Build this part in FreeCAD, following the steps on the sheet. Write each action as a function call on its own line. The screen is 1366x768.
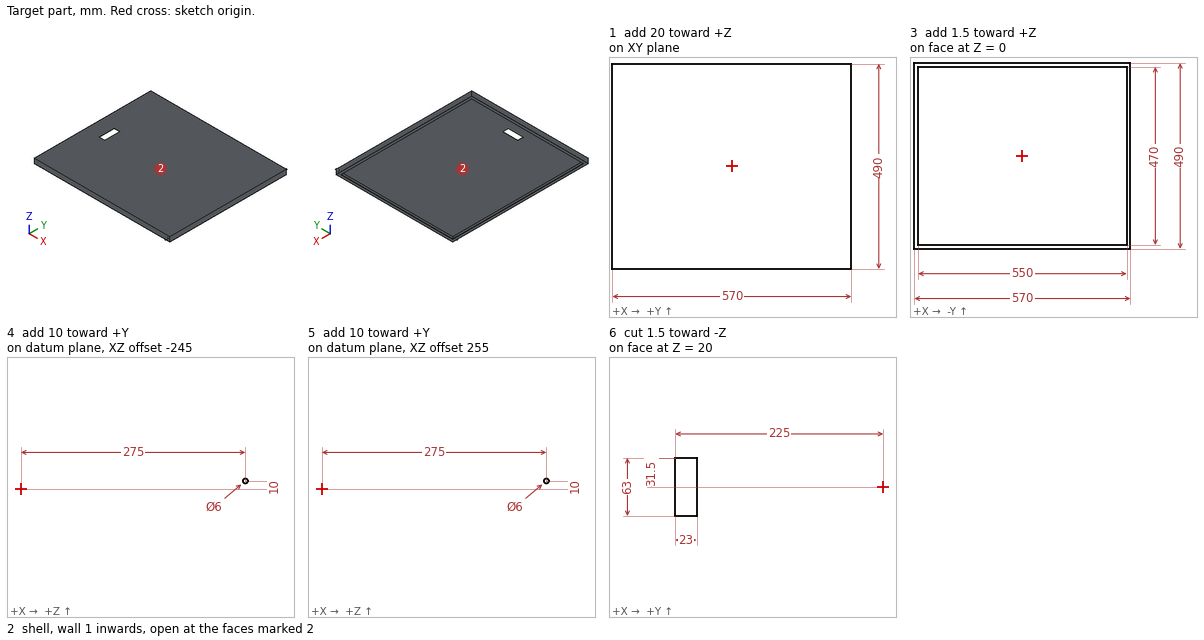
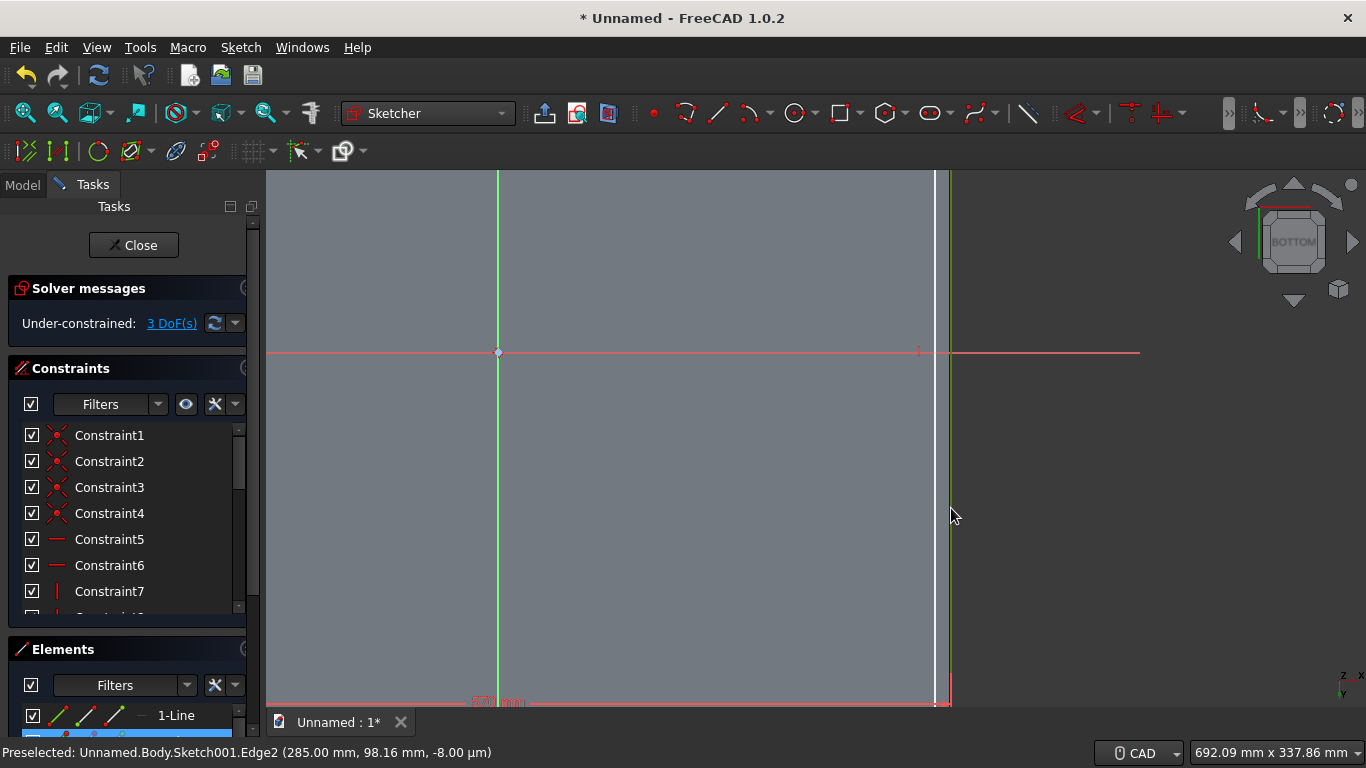
key(i)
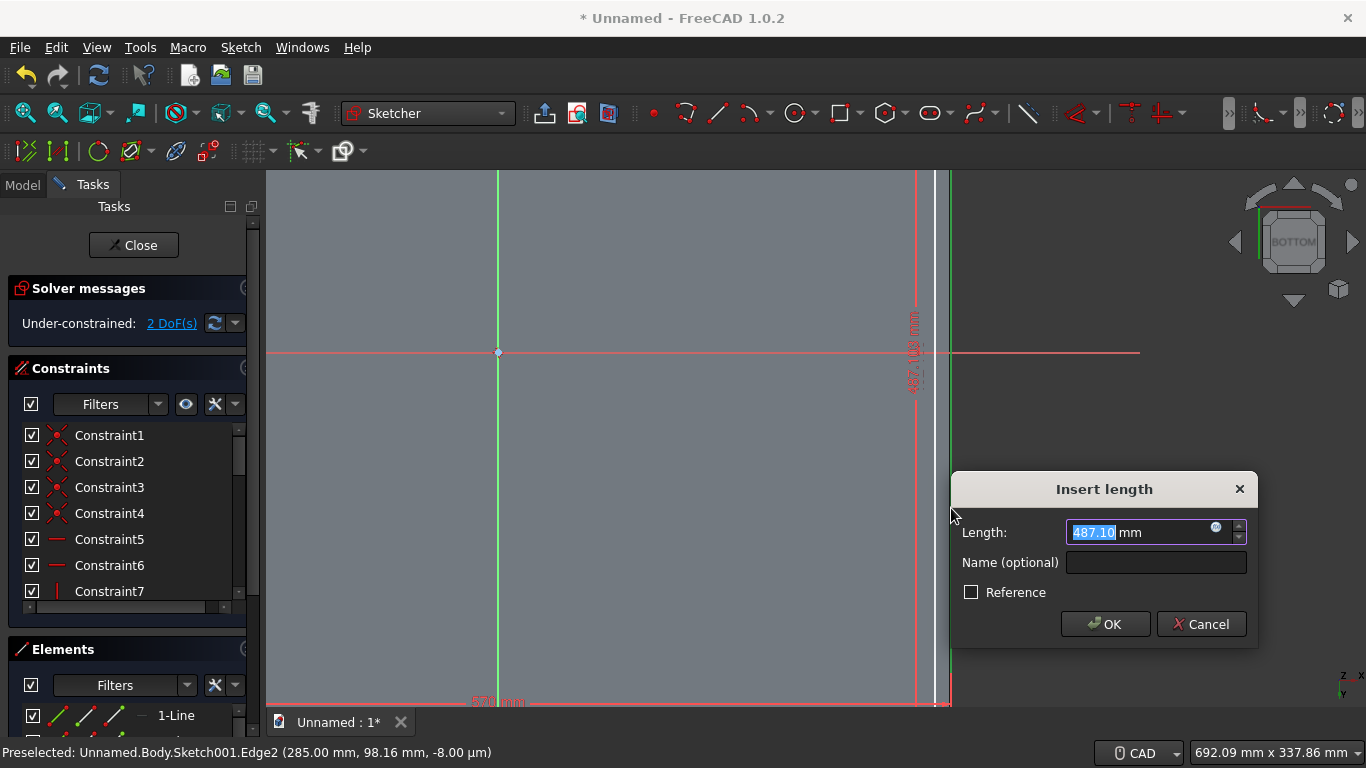
text(490)
key(Return)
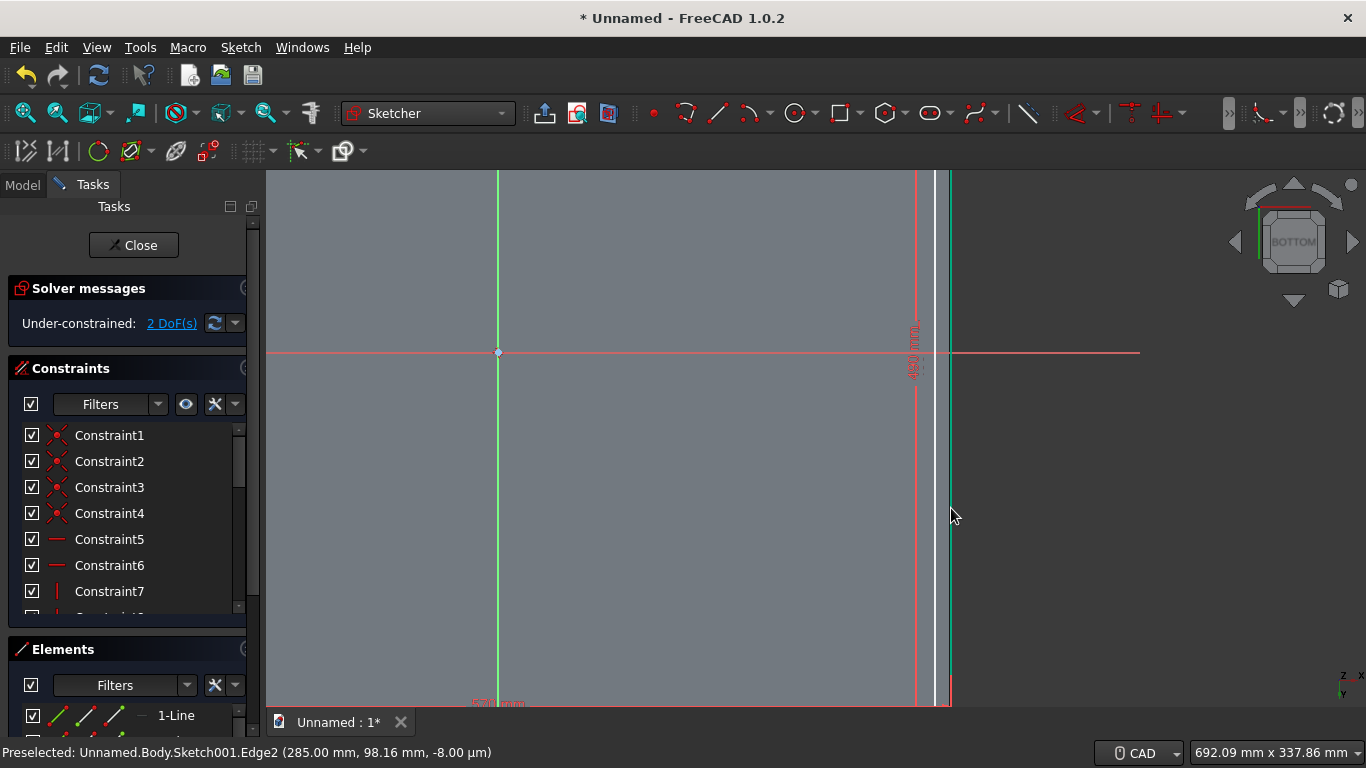
scroll(951, 508, down, 4)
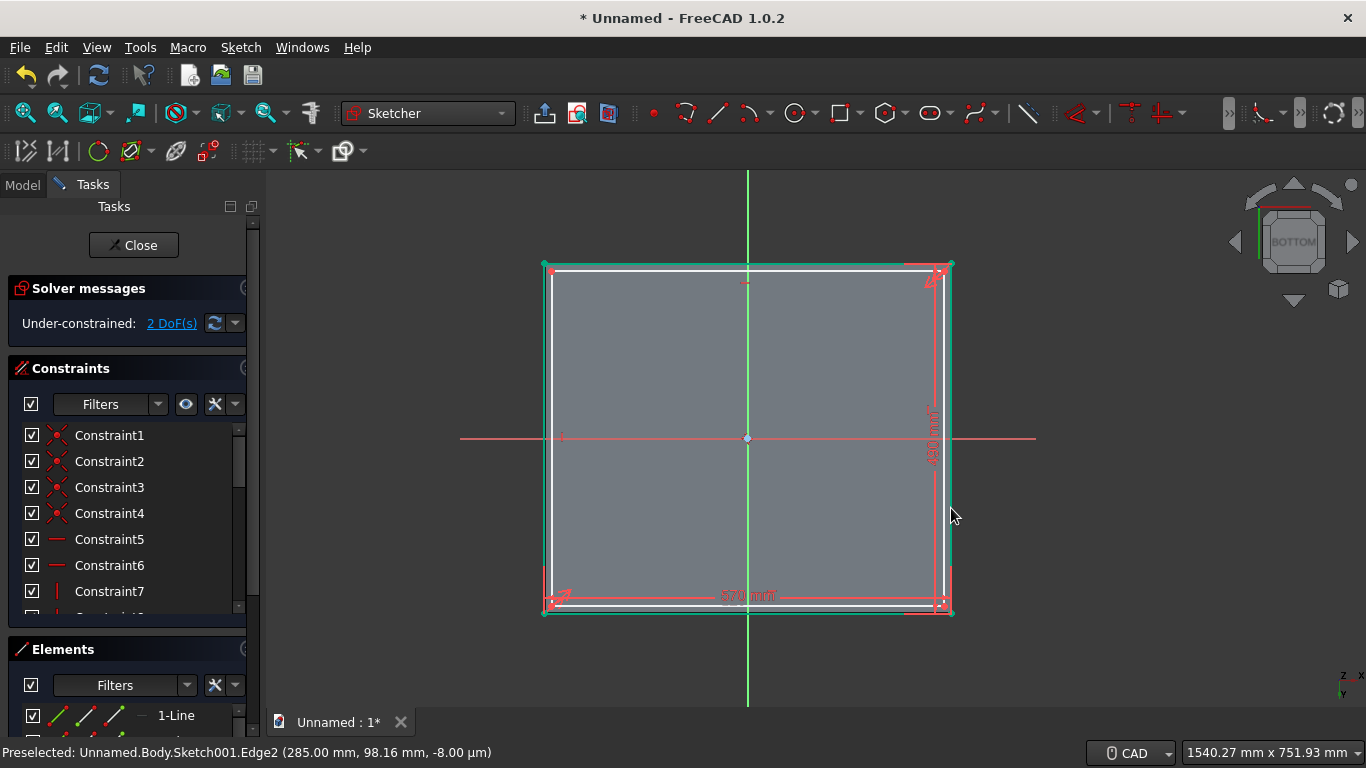
scroll(669, 606, up, 4)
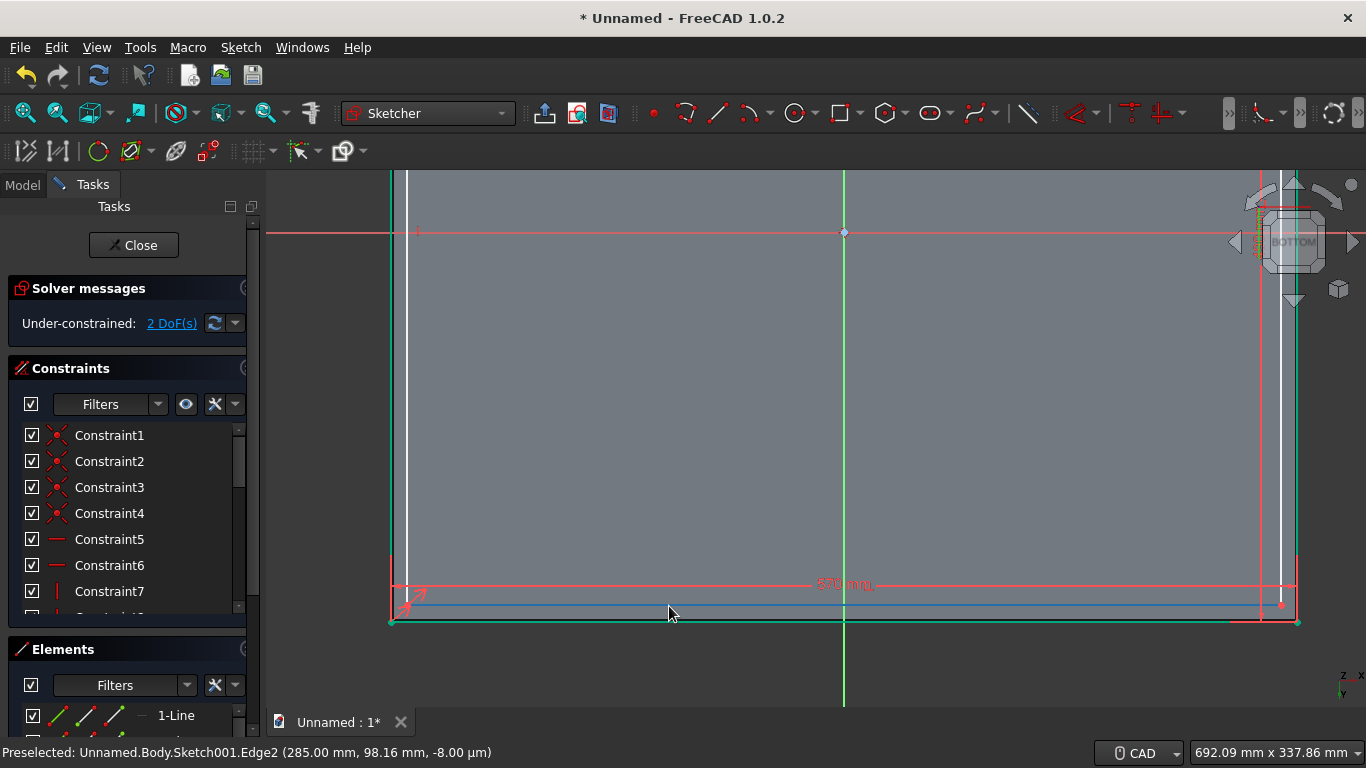
click(669, 605)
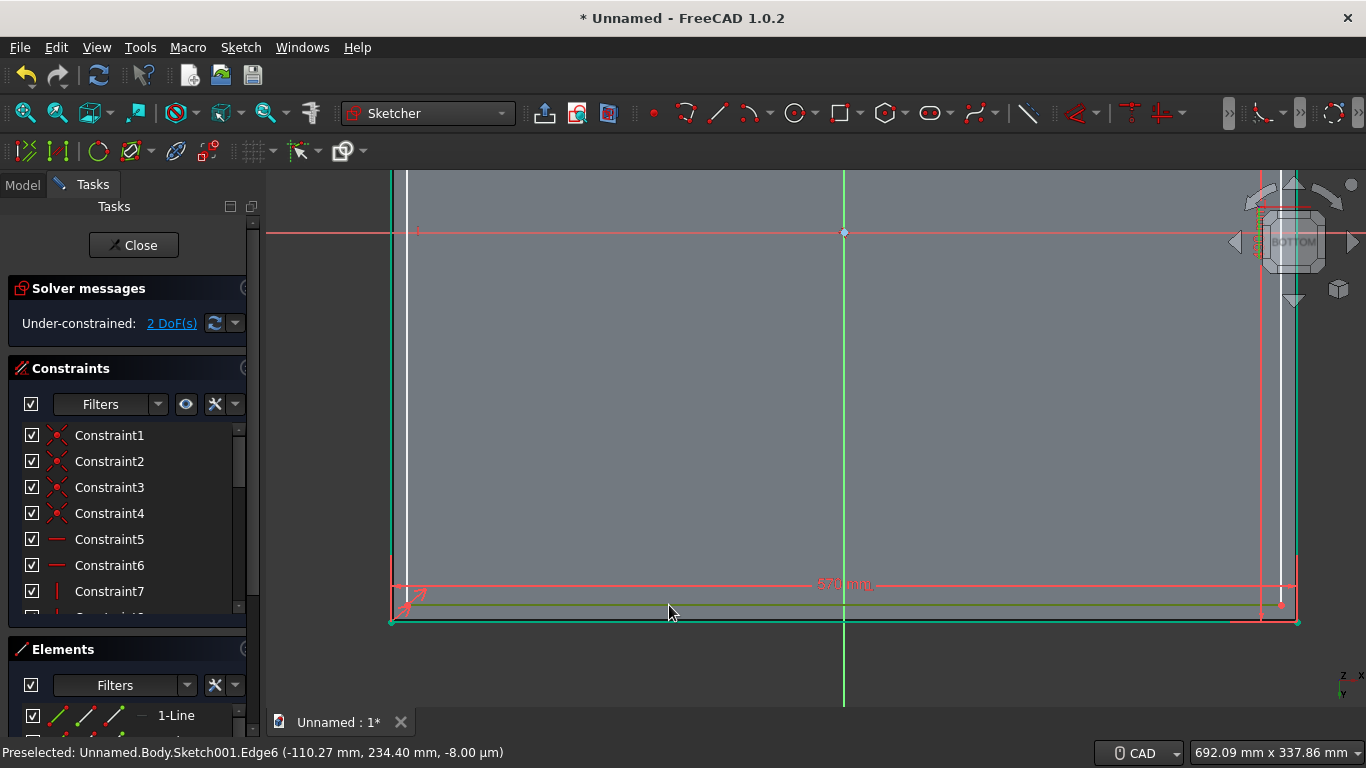
click(1098, 114)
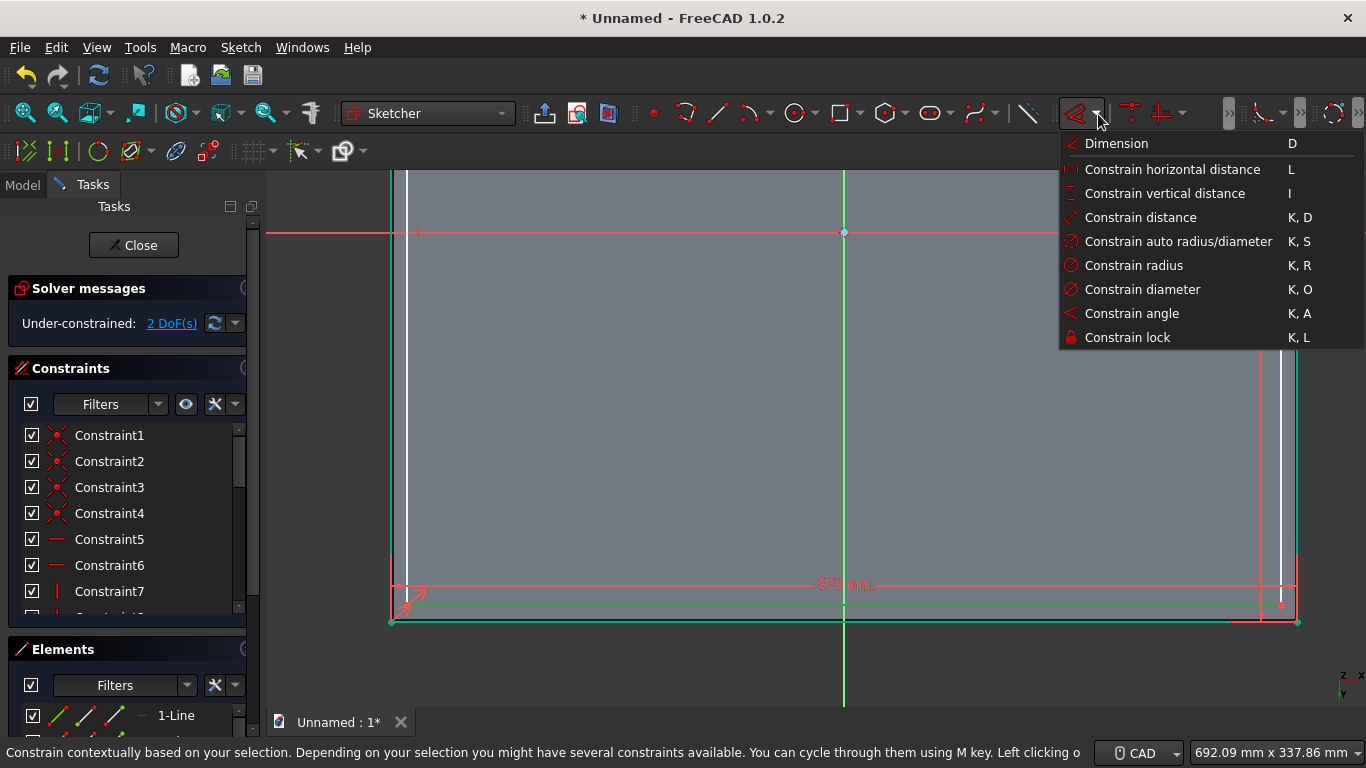
click(1212, 169)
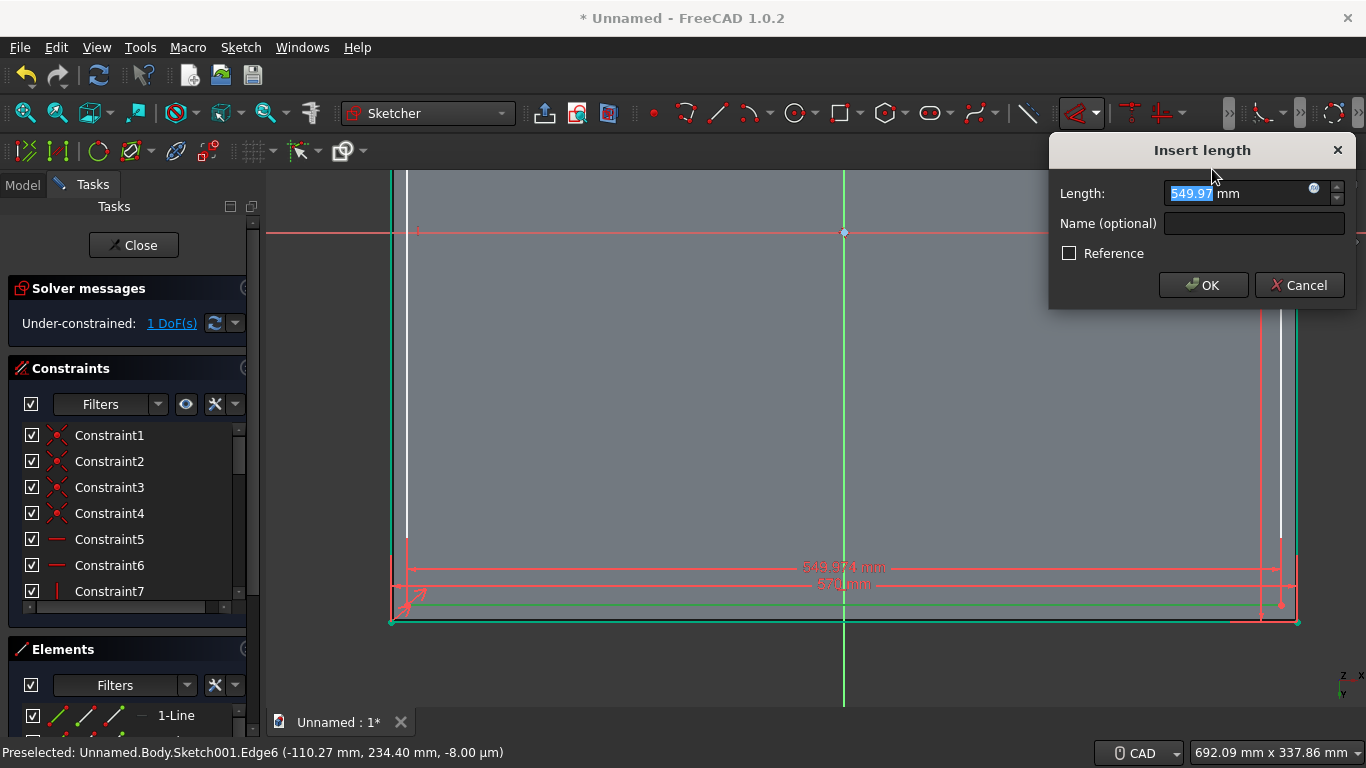
text(550)
key(Return)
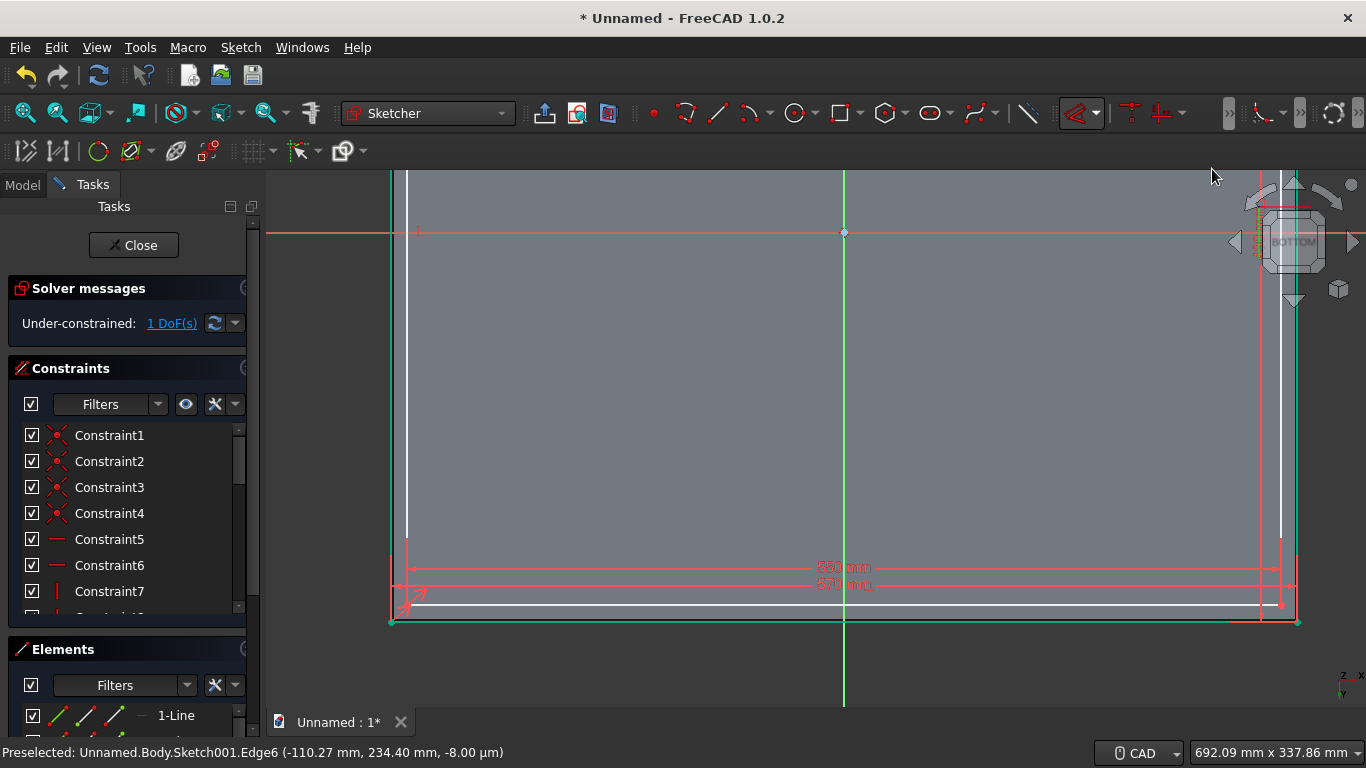
scroll(669, 606, down, 4)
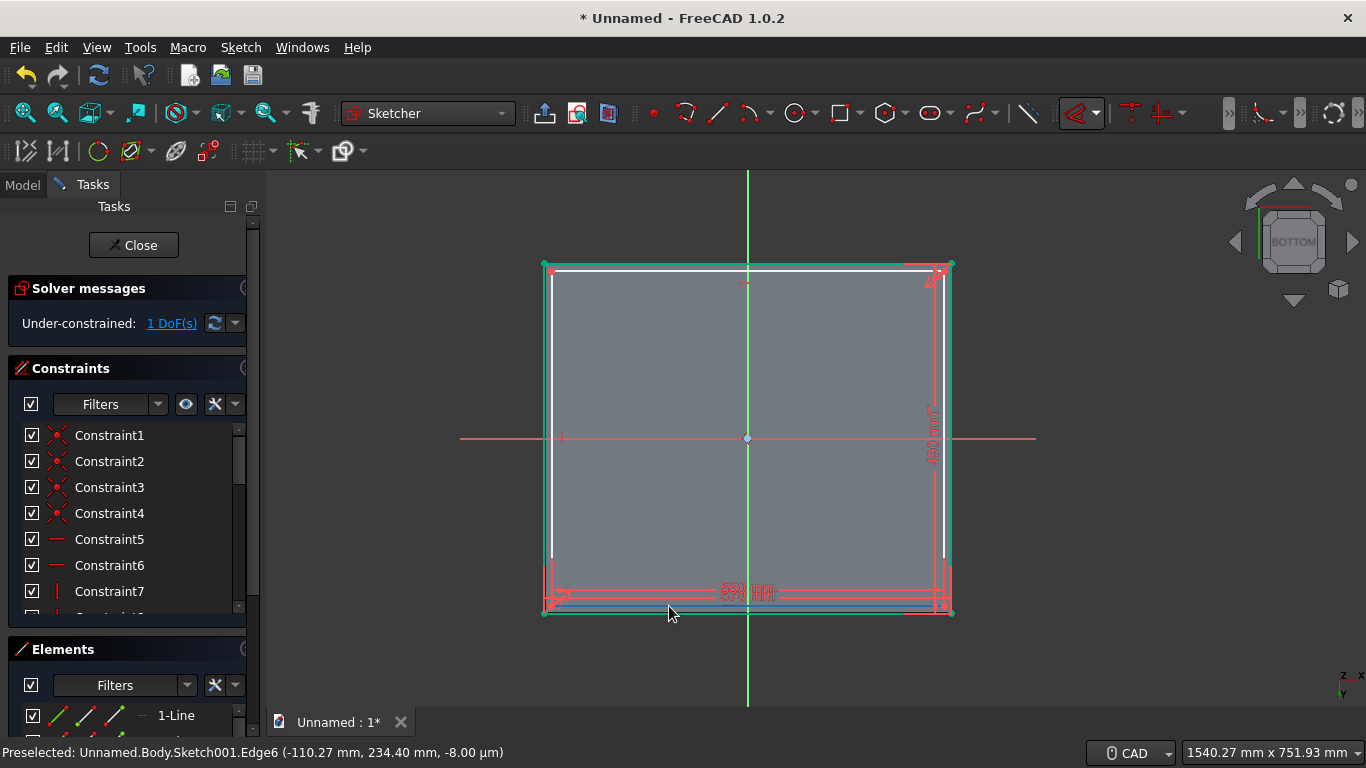
scroll(944, 506, up, 4)